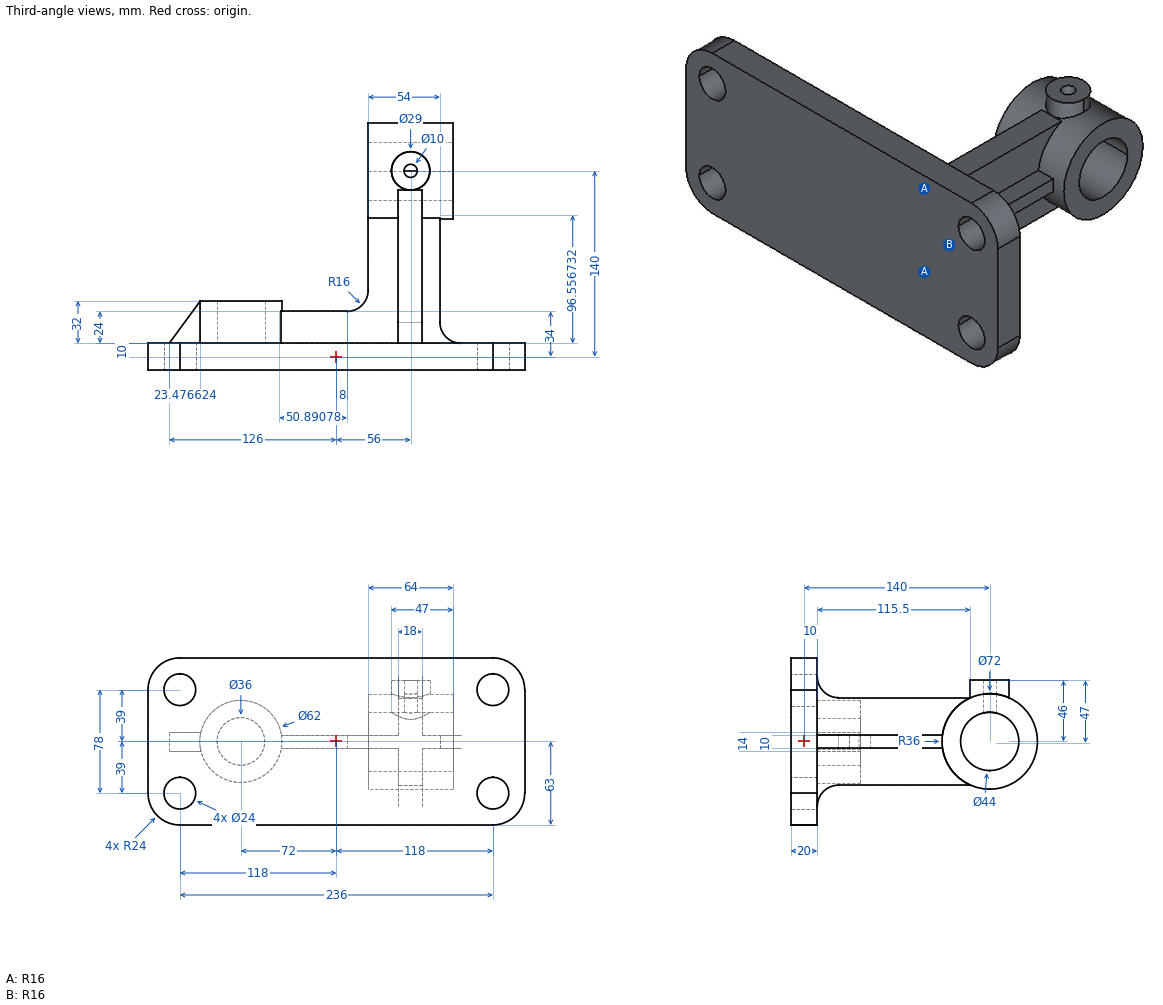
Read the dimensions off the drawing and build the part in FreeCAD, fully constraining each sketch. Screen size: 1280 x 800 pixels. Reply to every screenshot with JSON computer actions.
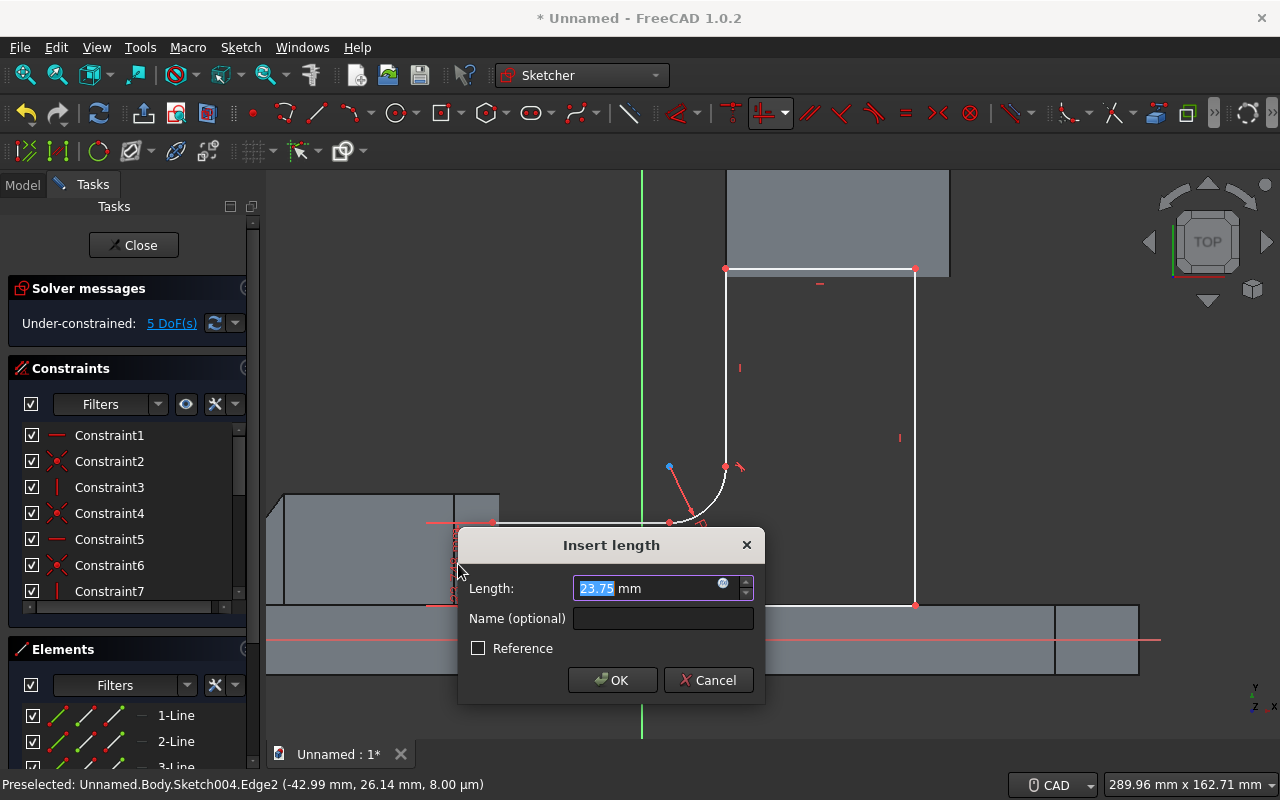
{"action": "type", "text": "24"}
{"action": "key", "text": "Return"}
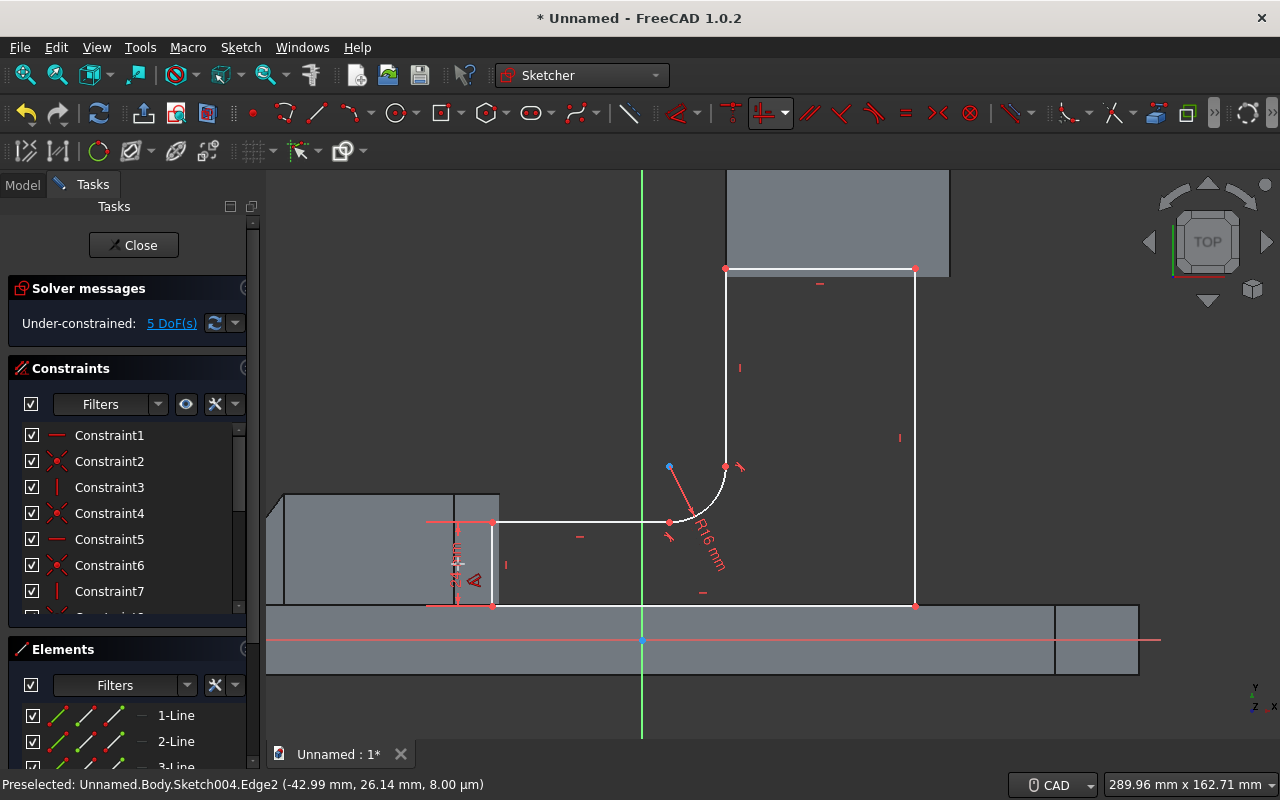
{"action": "left_click", "coordinate": [858, 269]}
{"action": "left_click", "coordinate": [820, 235]}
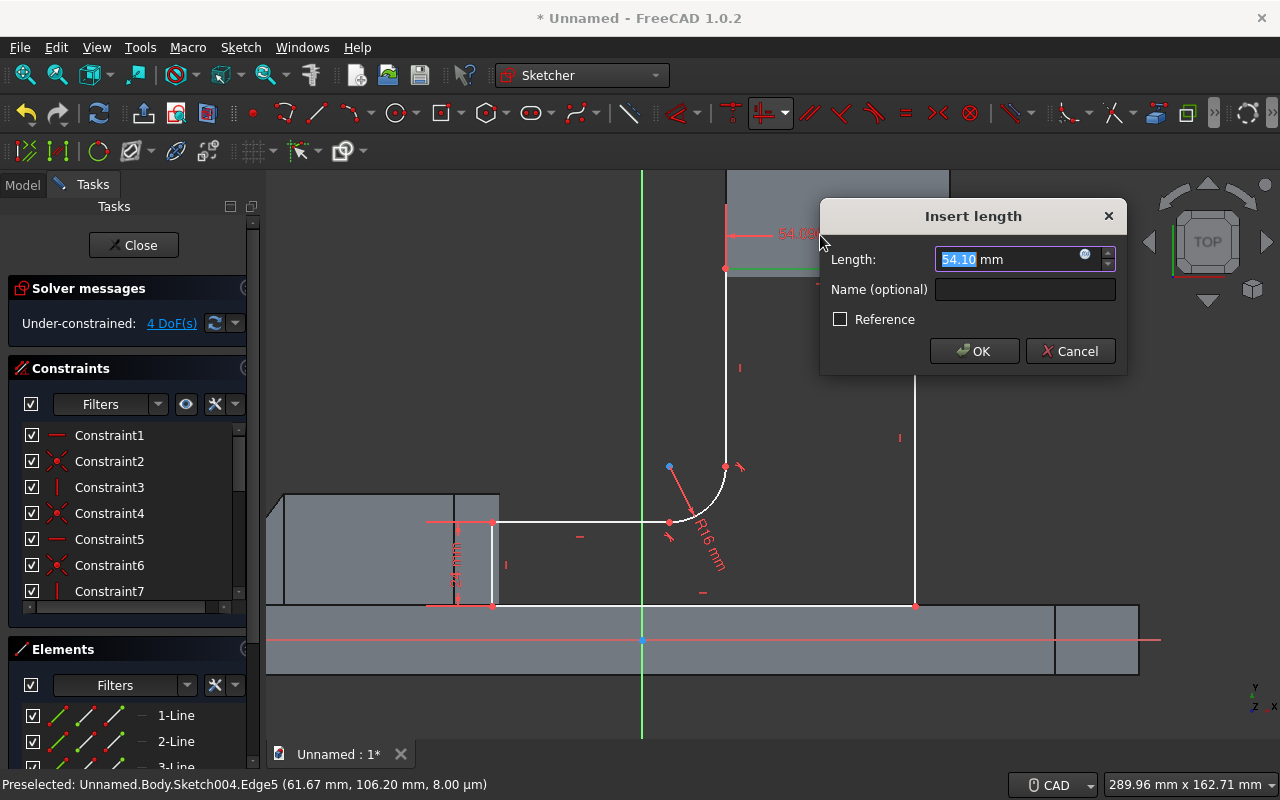
{"action": "type", "text": "54"}
{"action": "key", "text": "Return"}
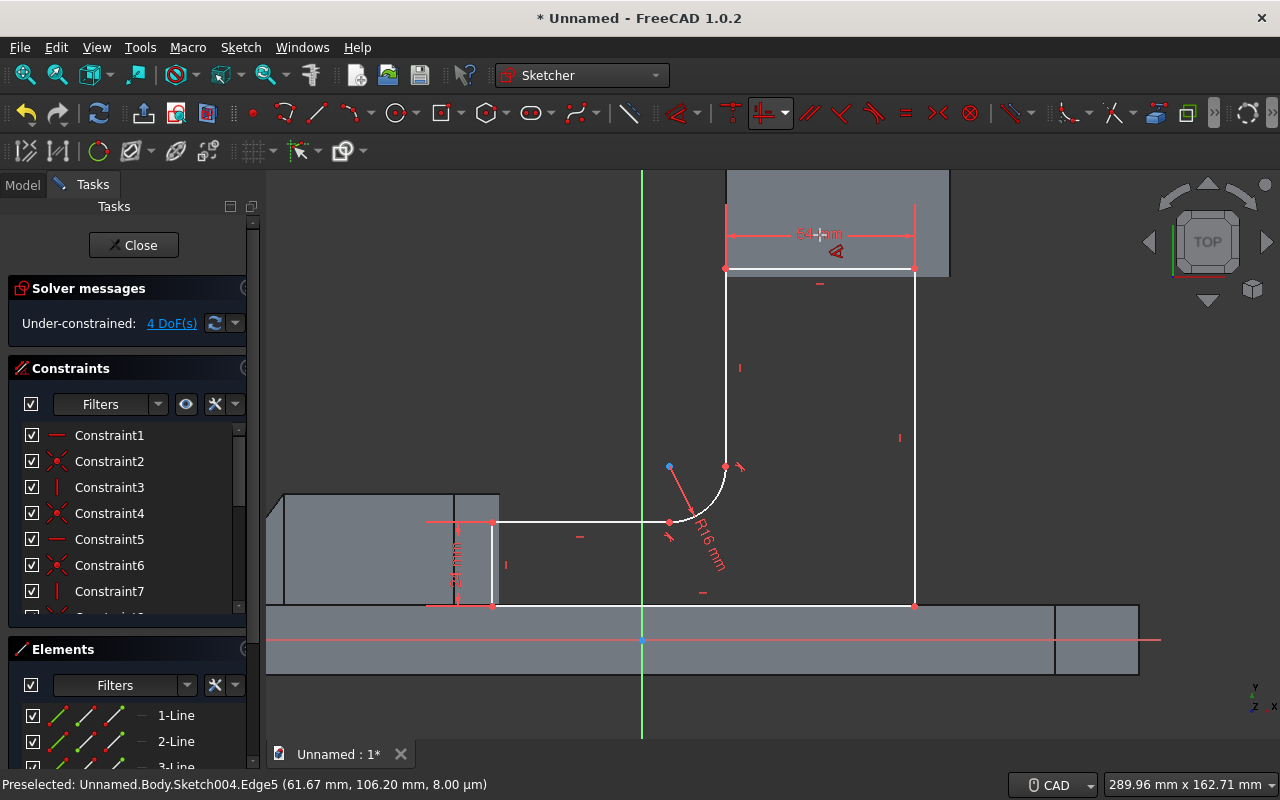
{"action": "scroll", "coordinate": [670, 522], "scroll_direction": "up", "scroll_amount": 2}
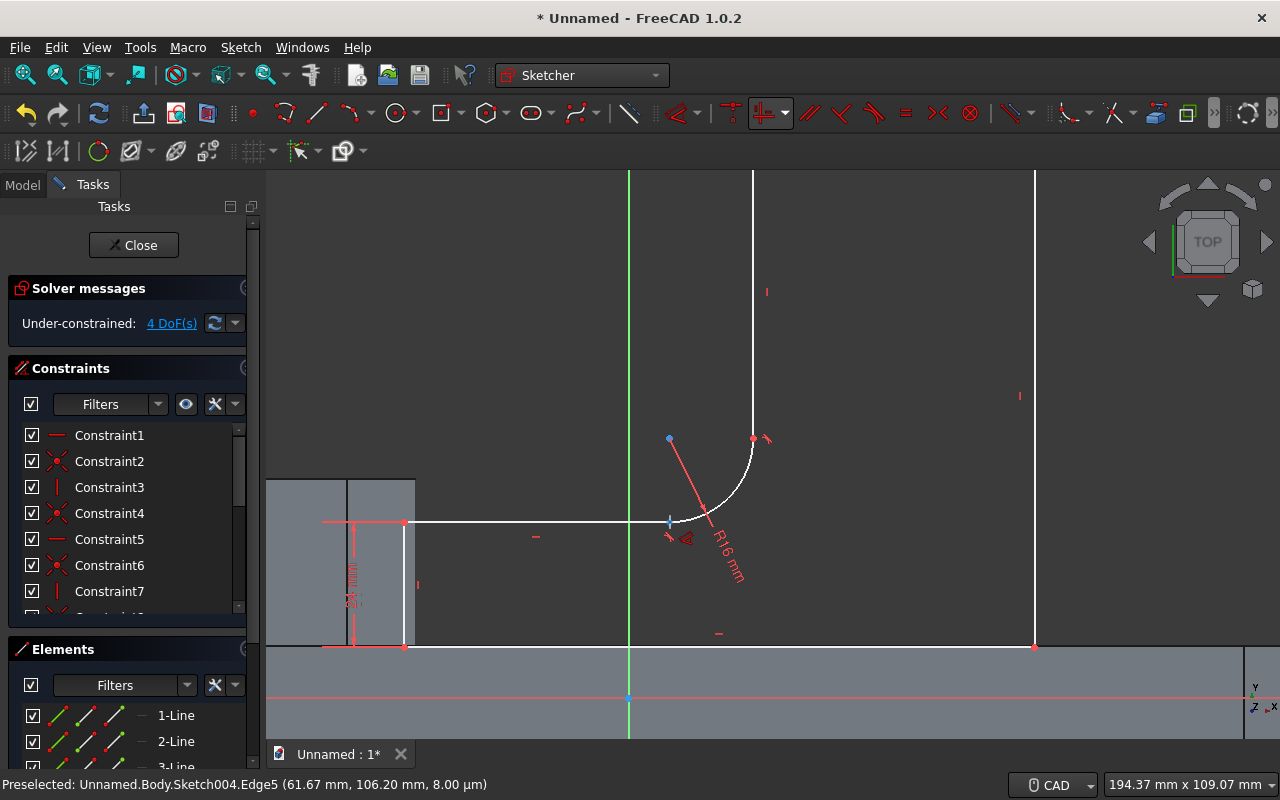
{"action": "left_click", "coordinate": [670, 522]}
{"action": "left_click", "coordinate": [649, 488]}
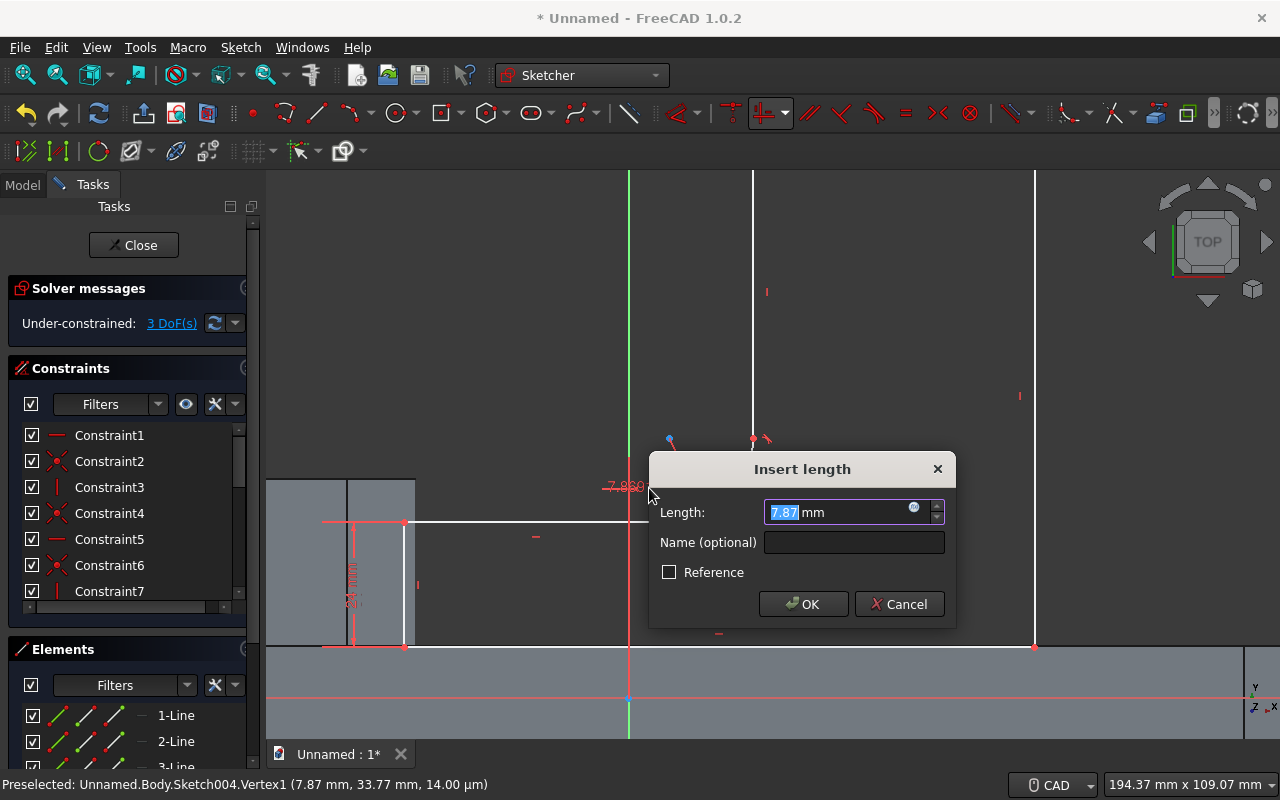
{"action": "type", "text": "8"}
{"action": "key", "text": "Return"}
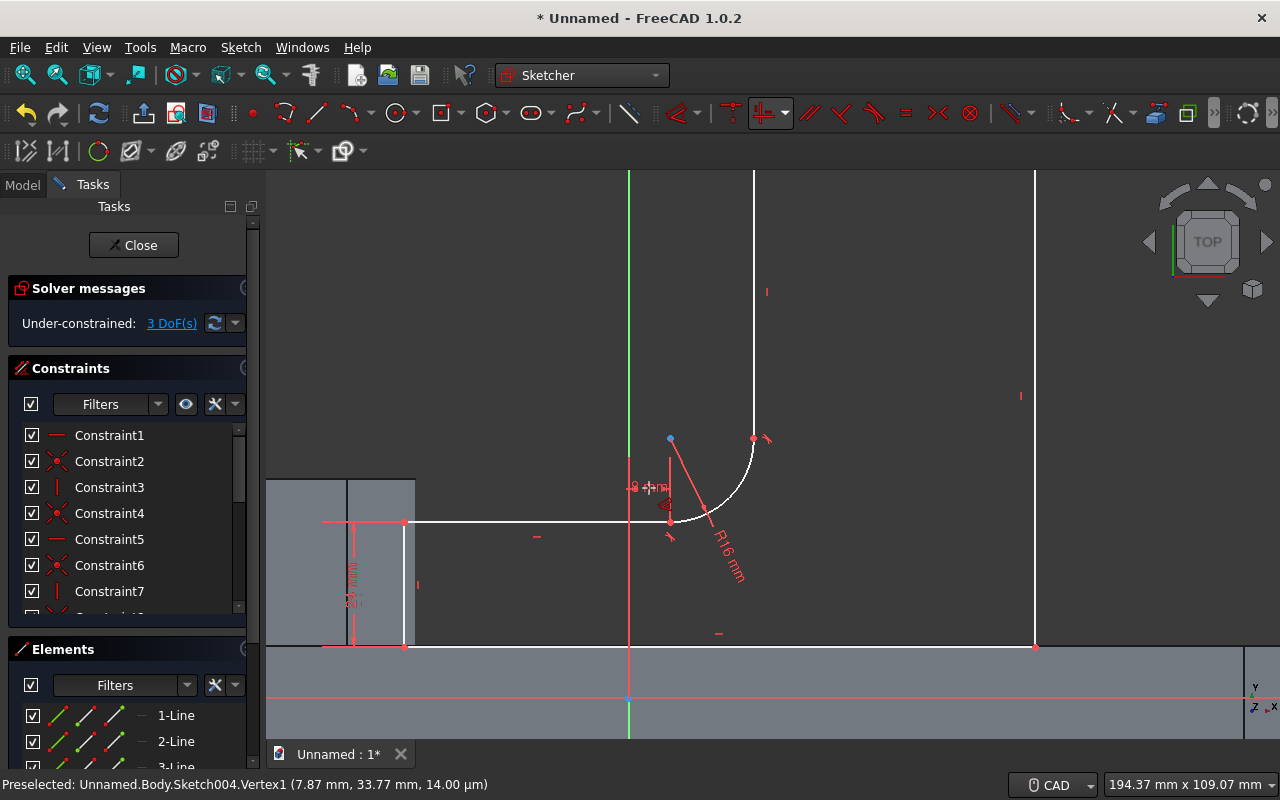
{"action": "left_click", "coordinate": [670, 522]}
{"action": "left_click", "coordinate": [595, 610]}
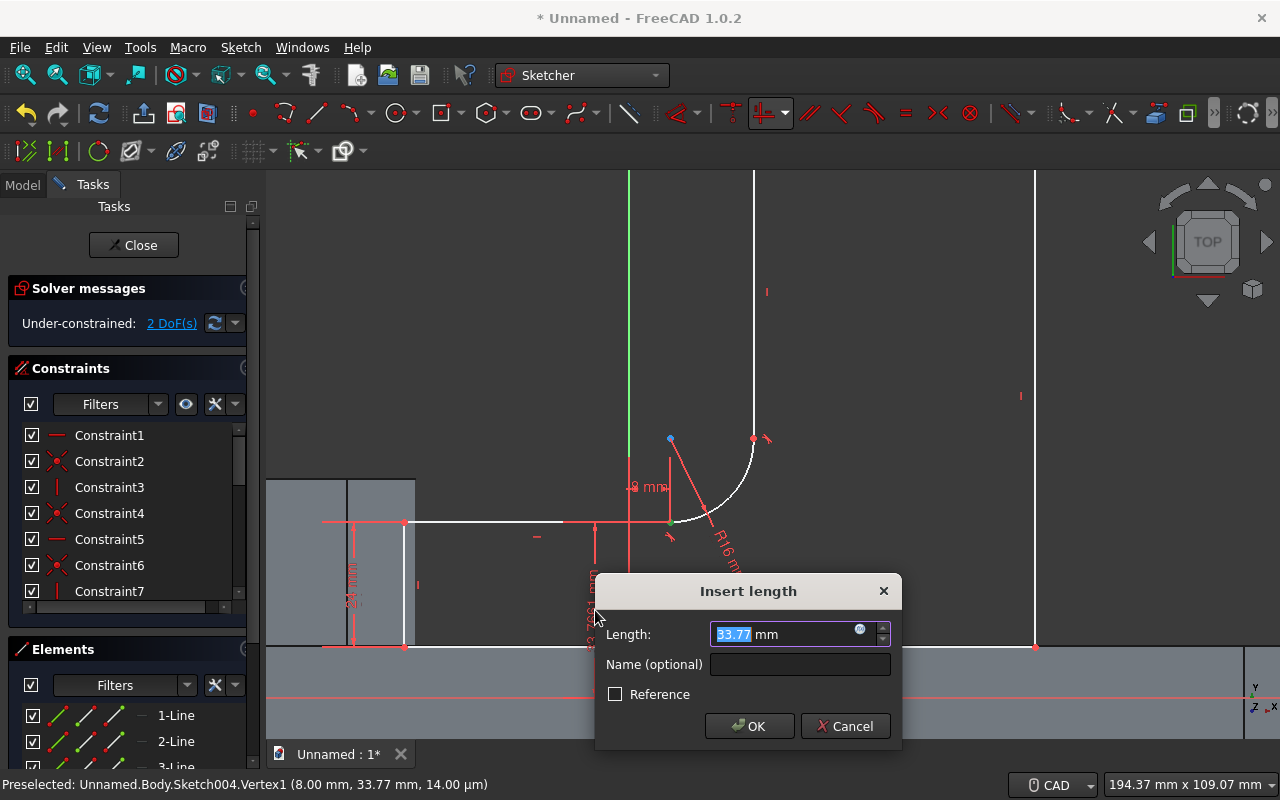
{"action": "type", "text": "34"}
{"action": "key", "text": "Return"}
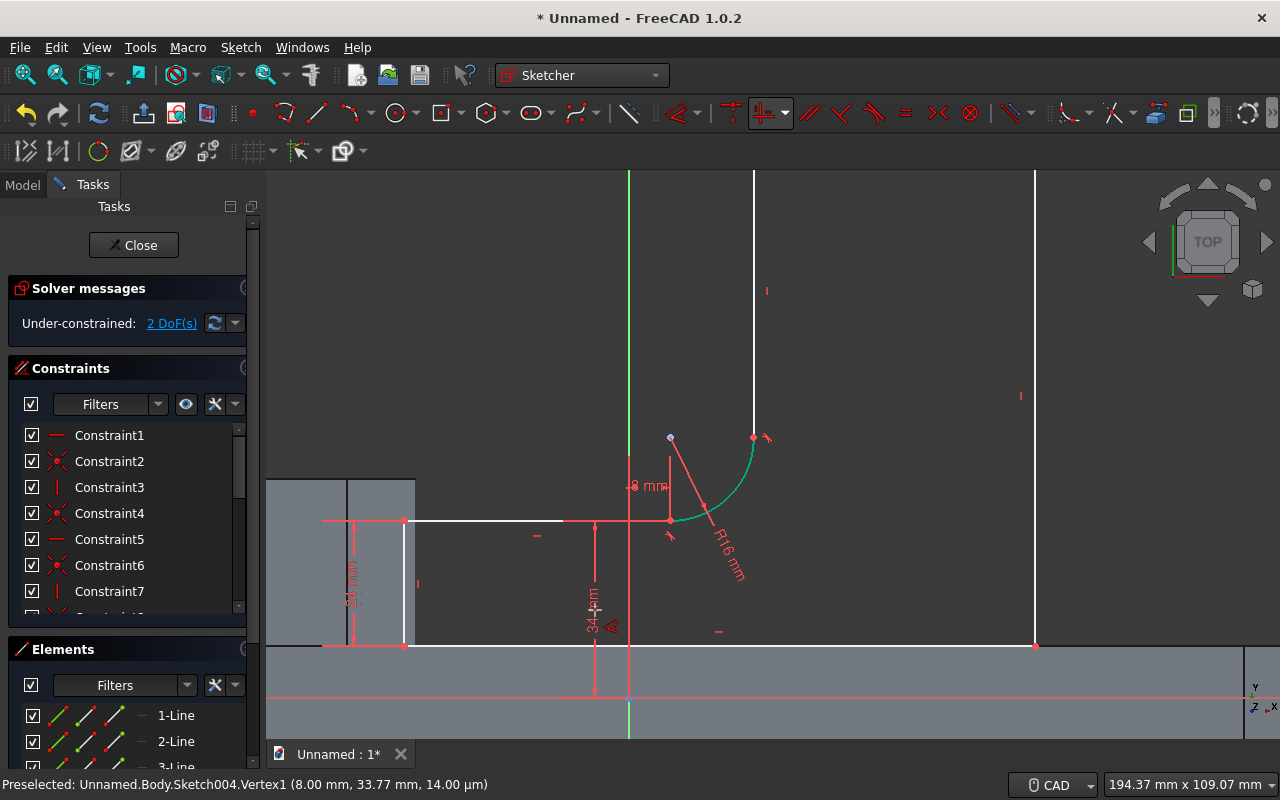
{"action": "left_click", "coordinate": [590, 521]}
{"action": "left_click", "coordinate": [537, 555]}